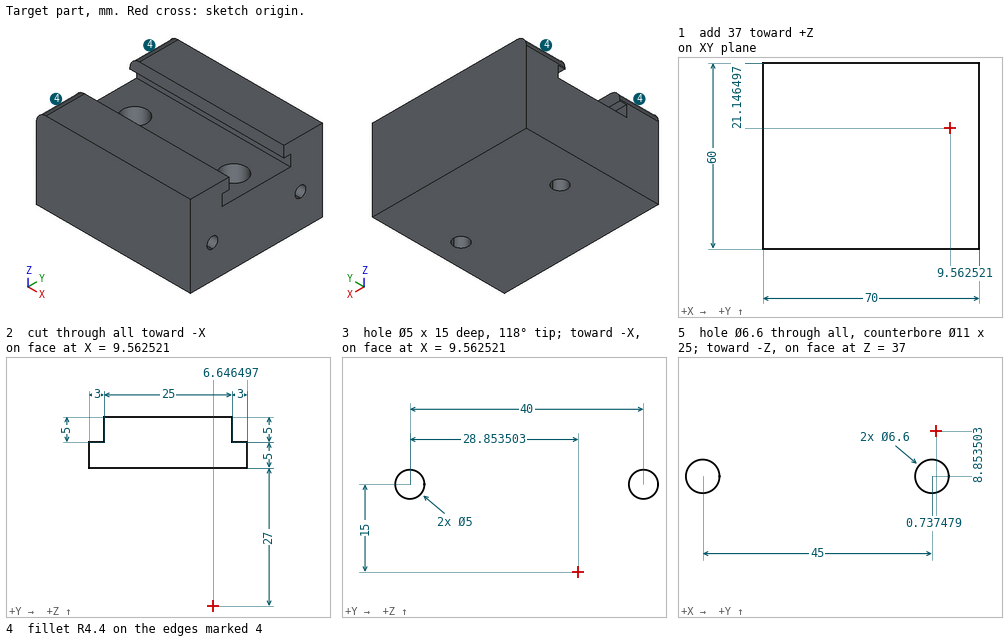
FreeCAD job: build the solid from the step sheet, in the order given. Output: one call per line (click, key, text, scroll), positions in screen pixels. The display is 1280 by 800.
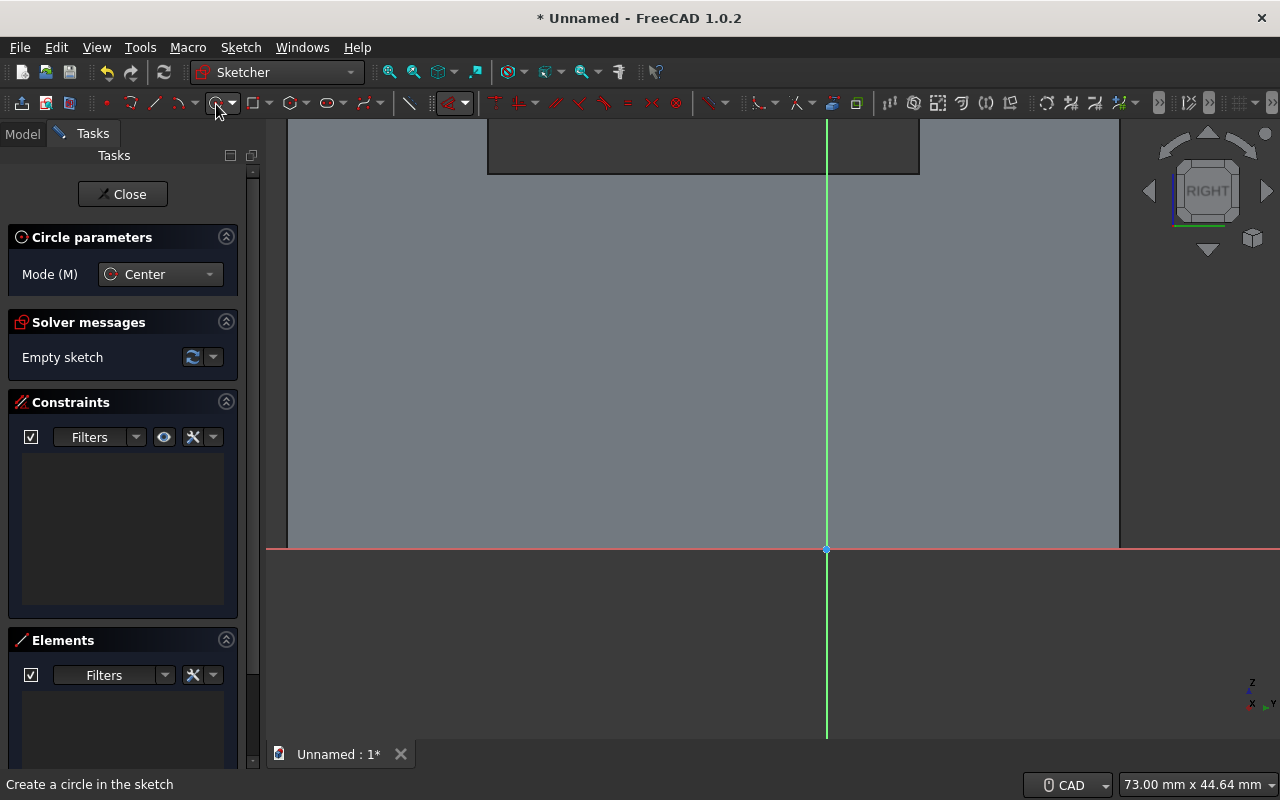
click(426, 341)
click(450, 316)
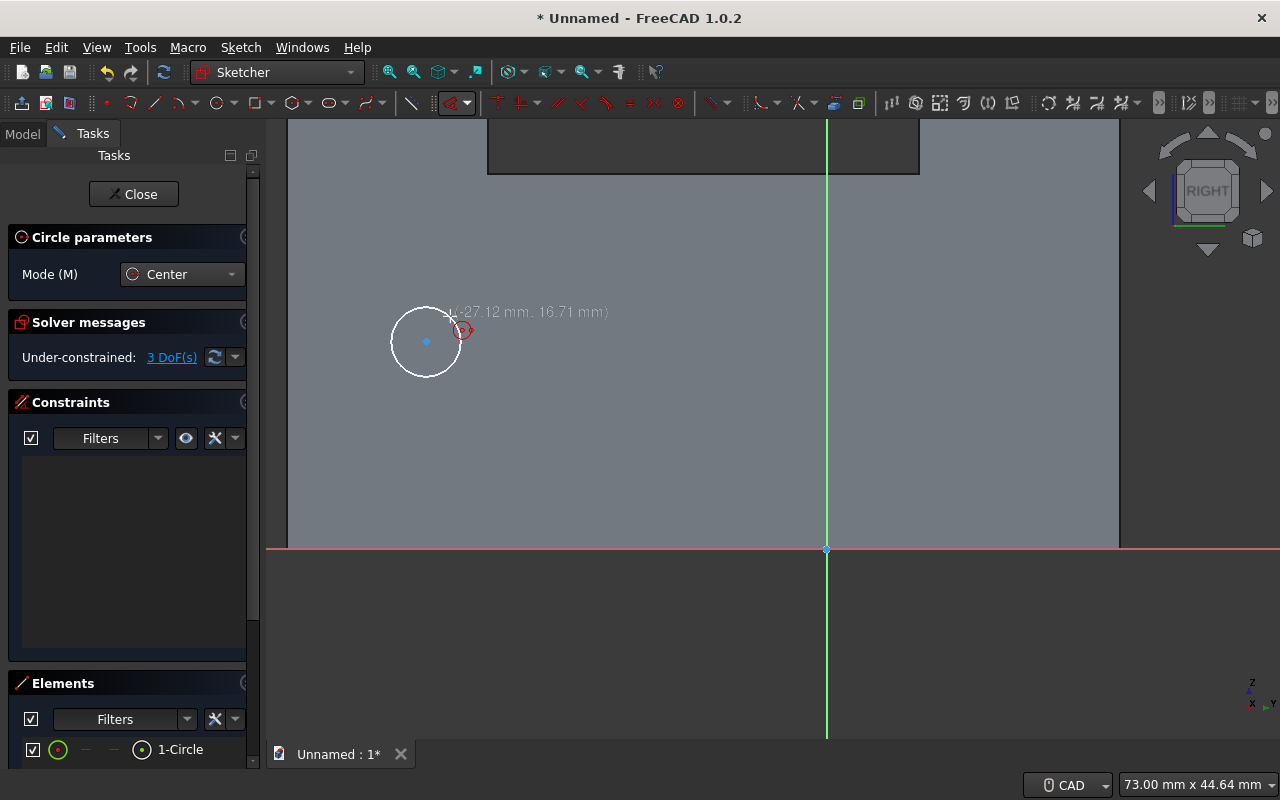
click(981, 341)
click(1006, 316)
key(Escape)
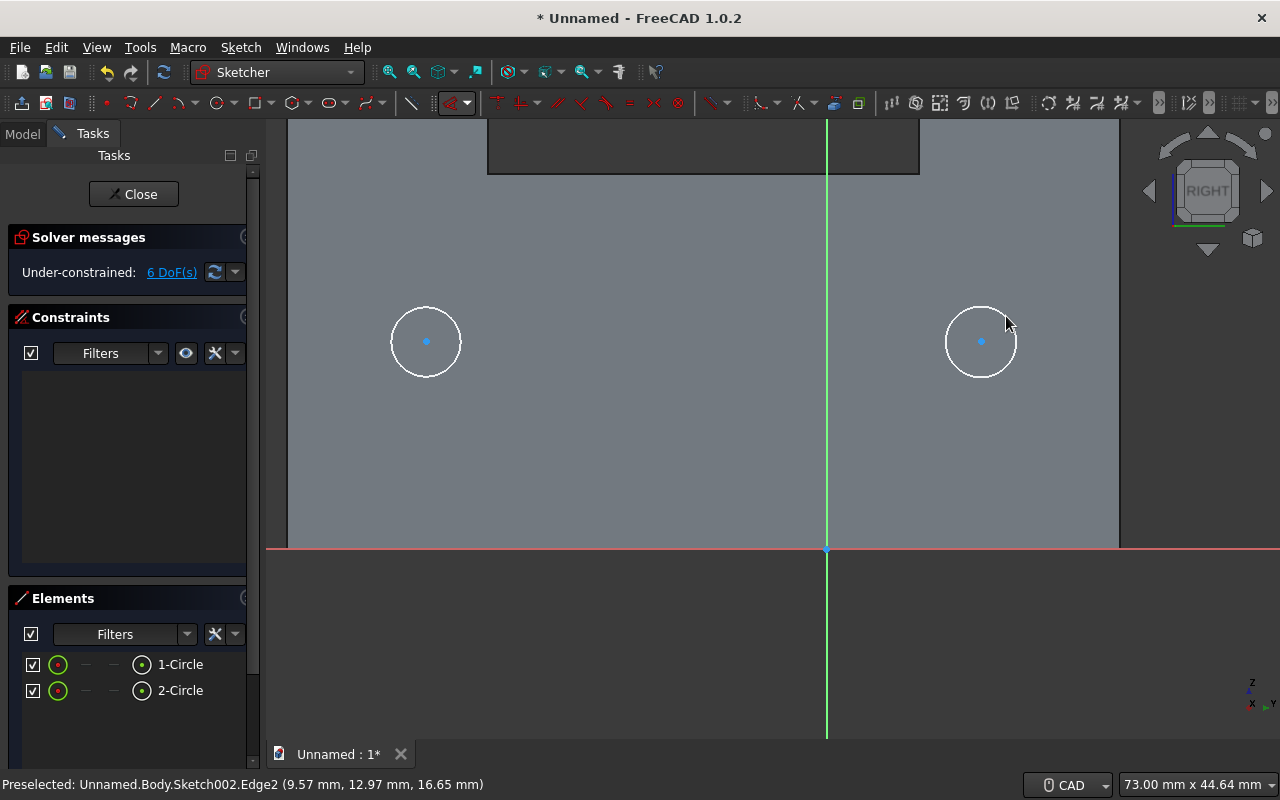
click(450, 317)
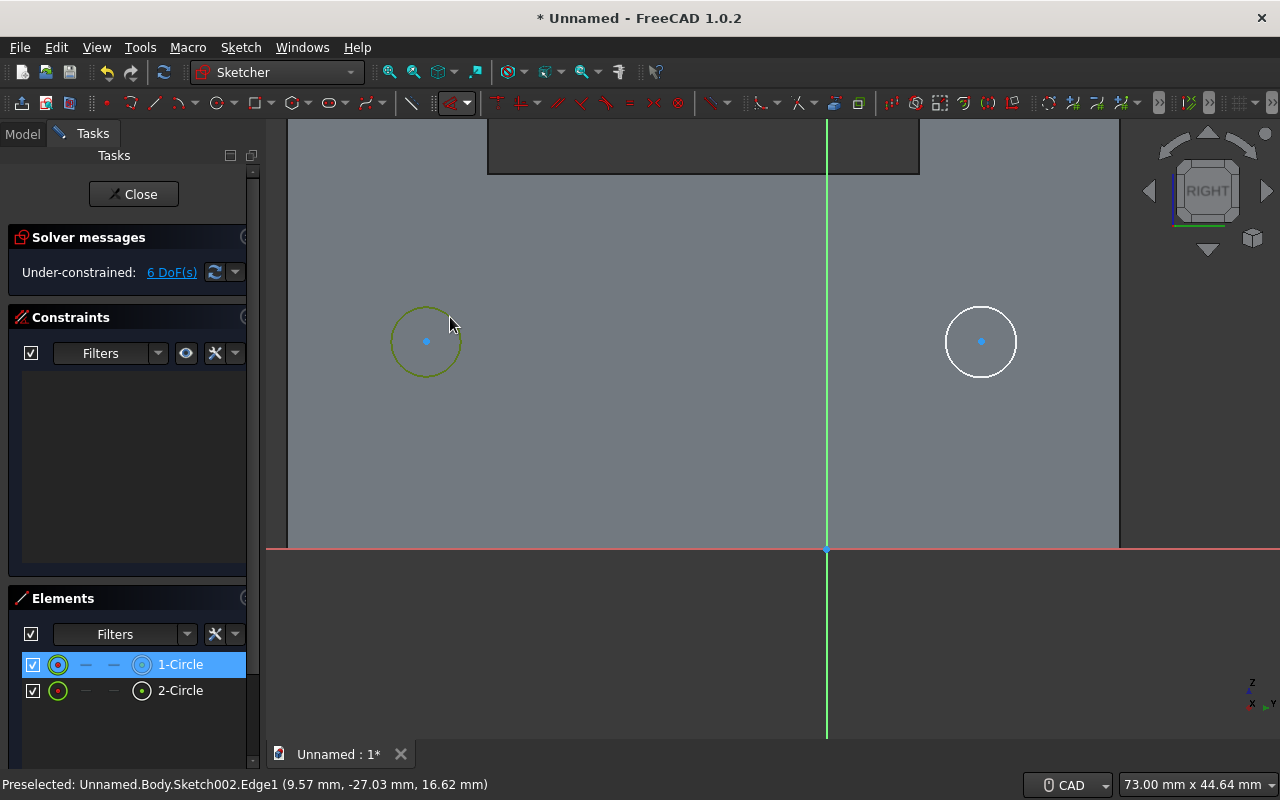
click(1006, 317)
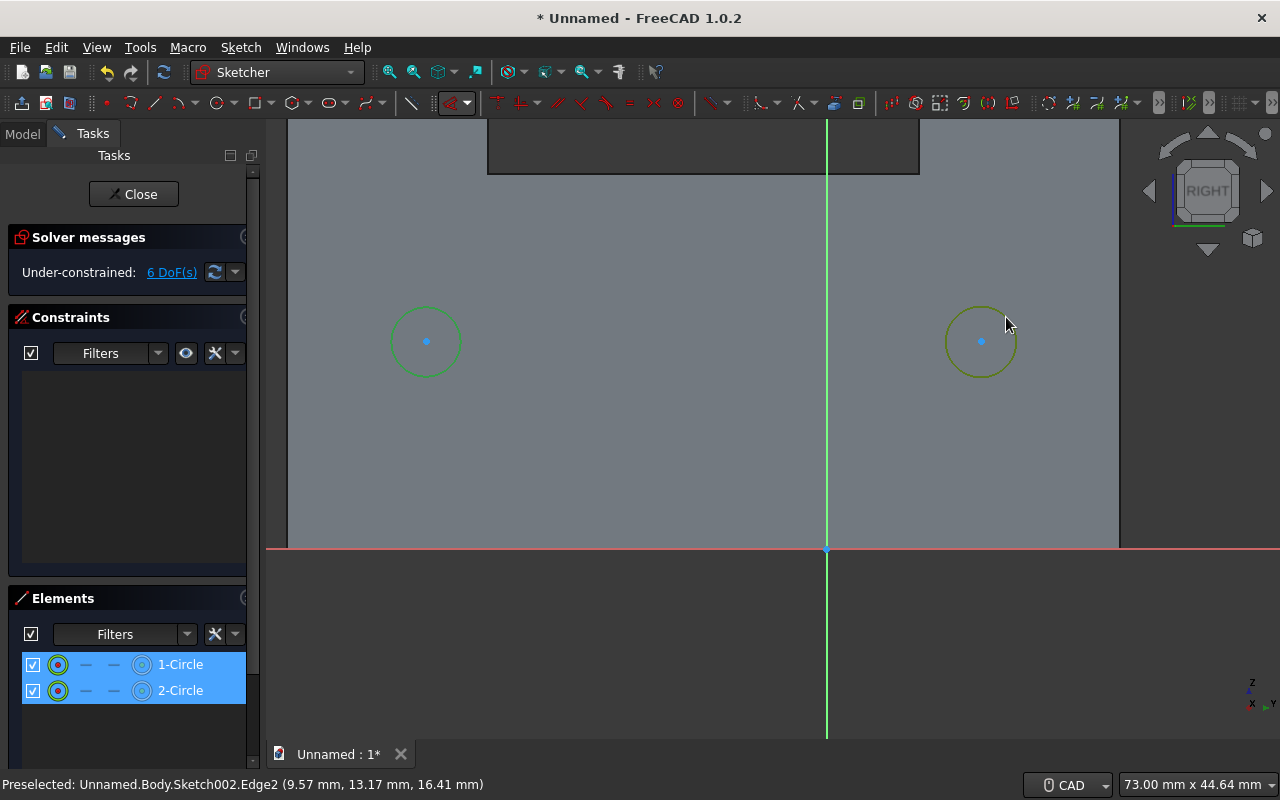
click(630, 104)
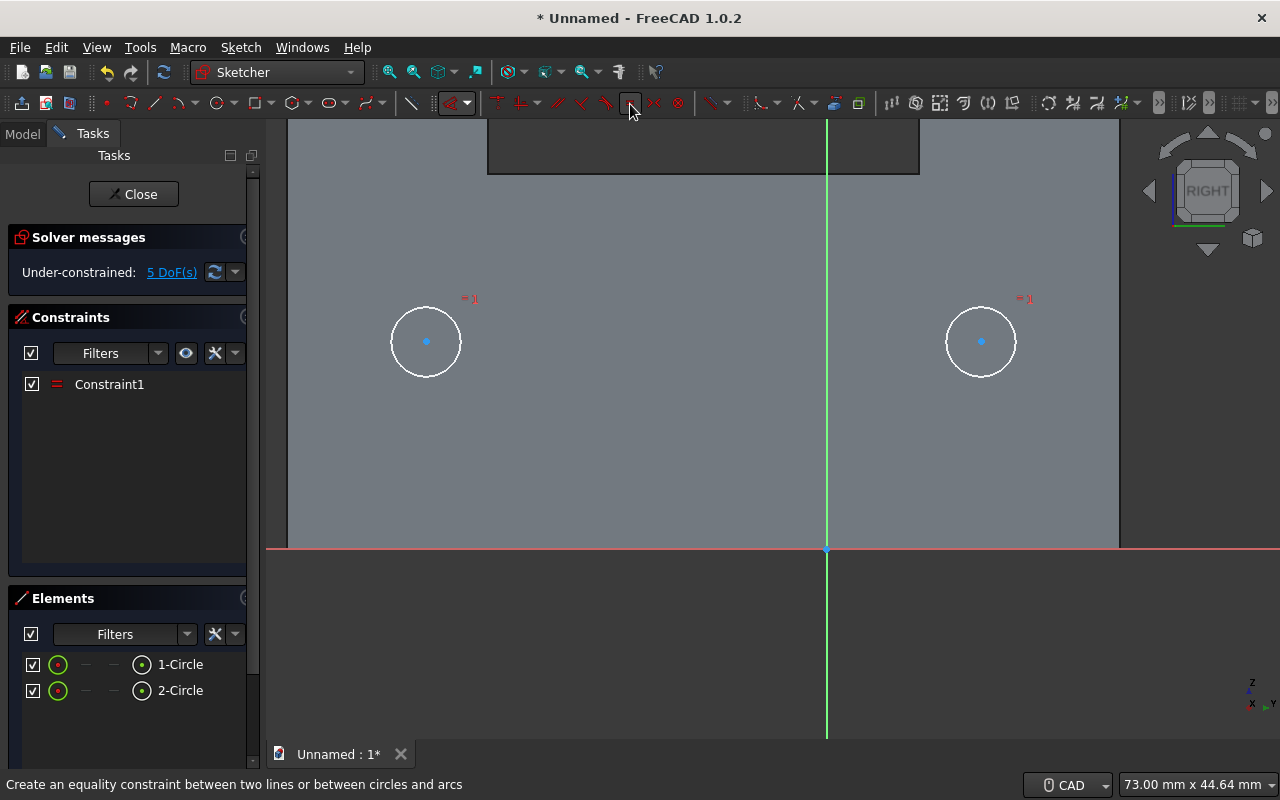
click(426, 342)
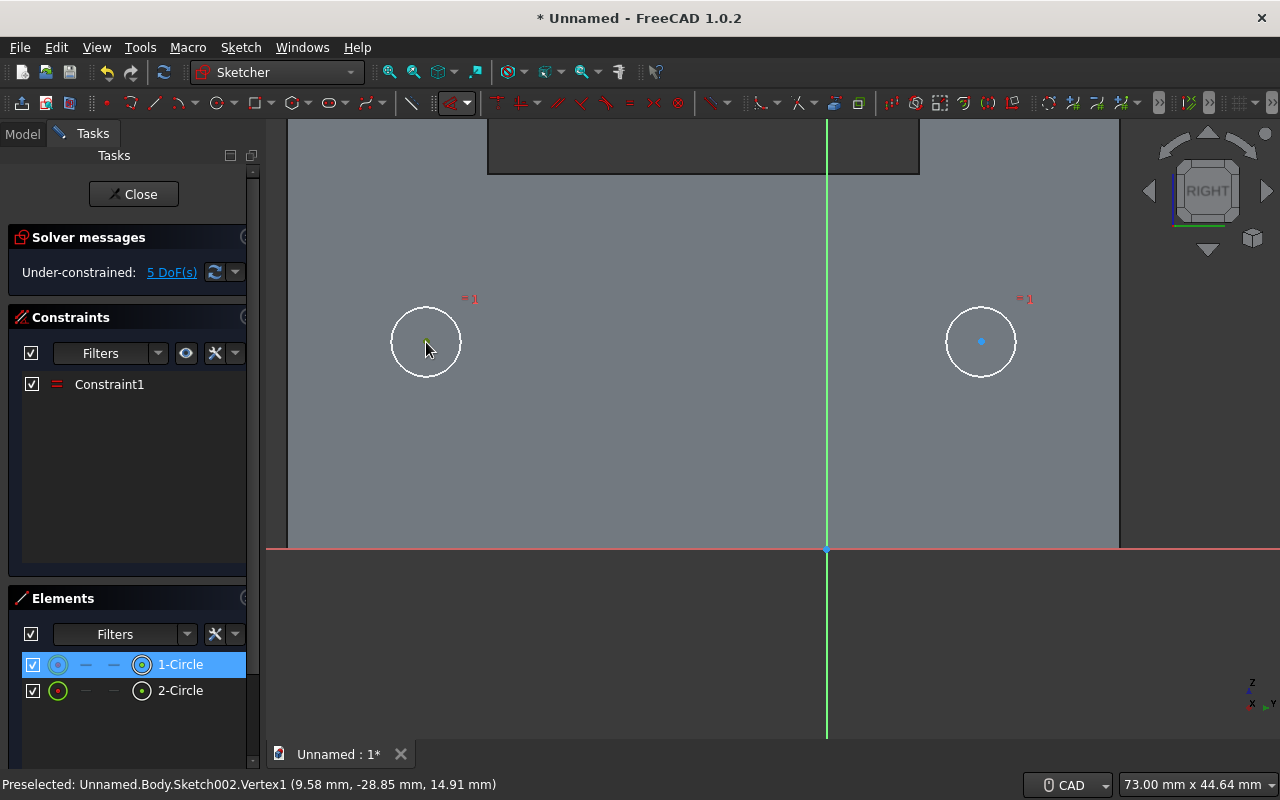
click(981, 342)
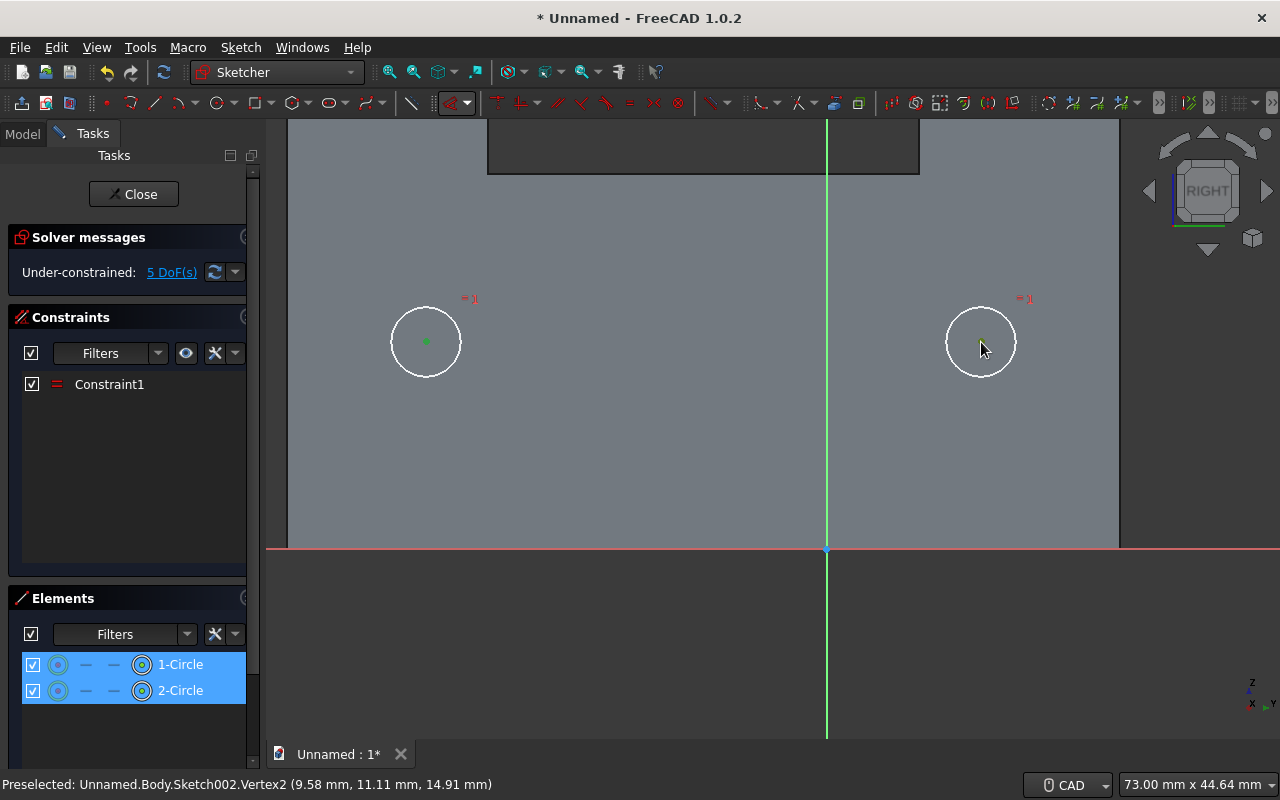
key(h)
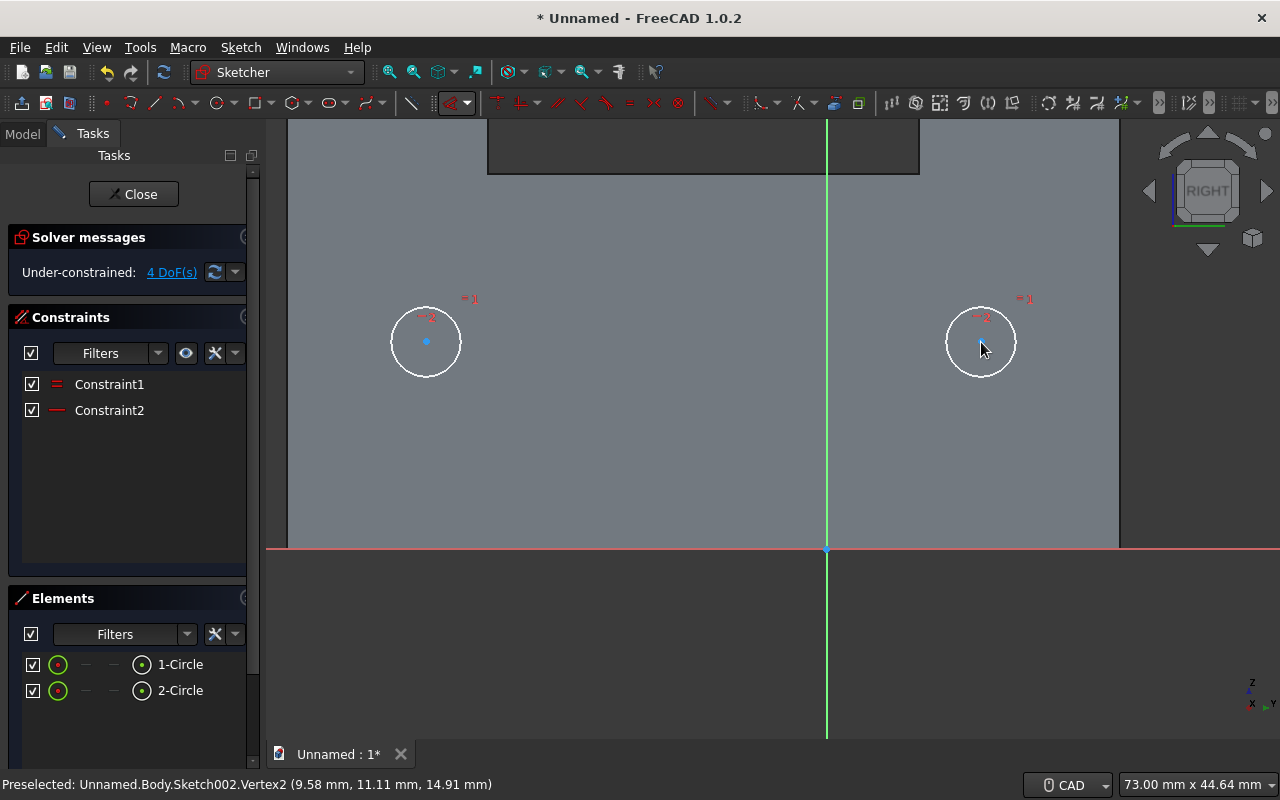
click(450, 317)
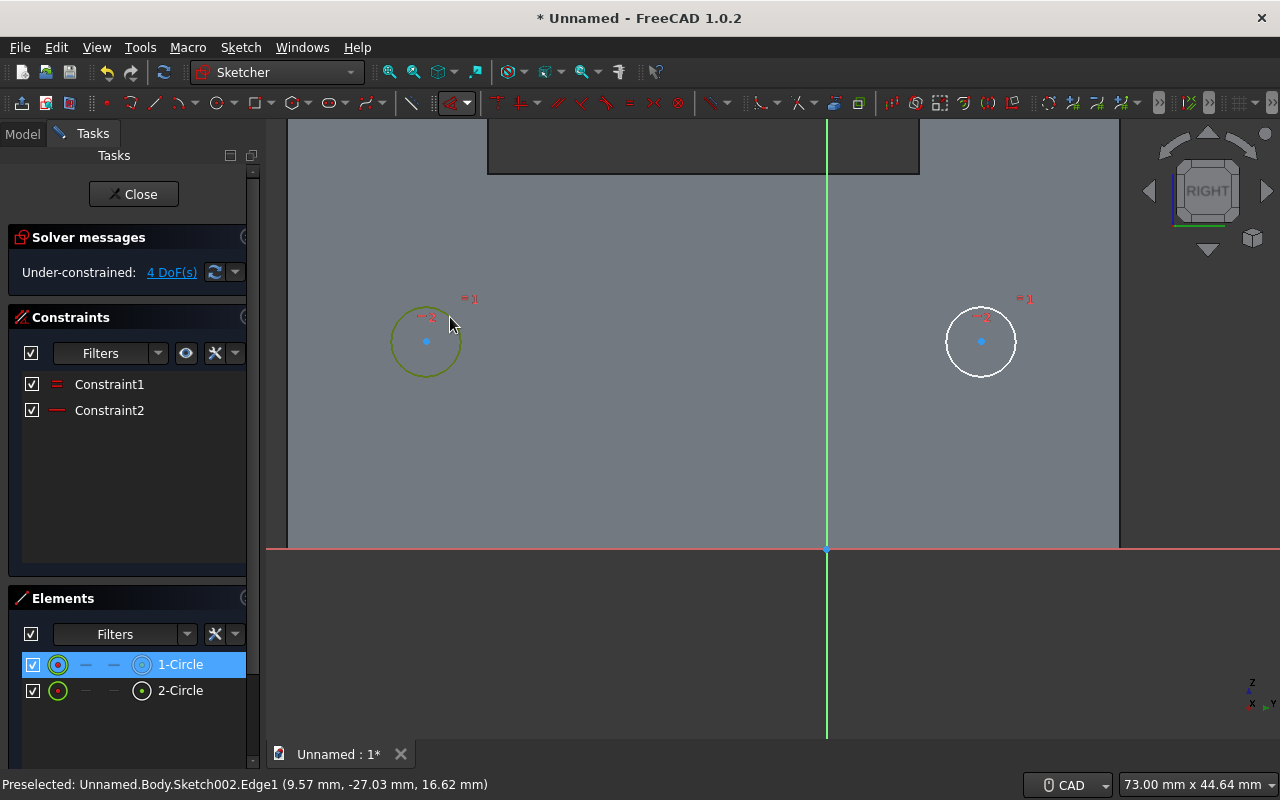
click(470, 104)